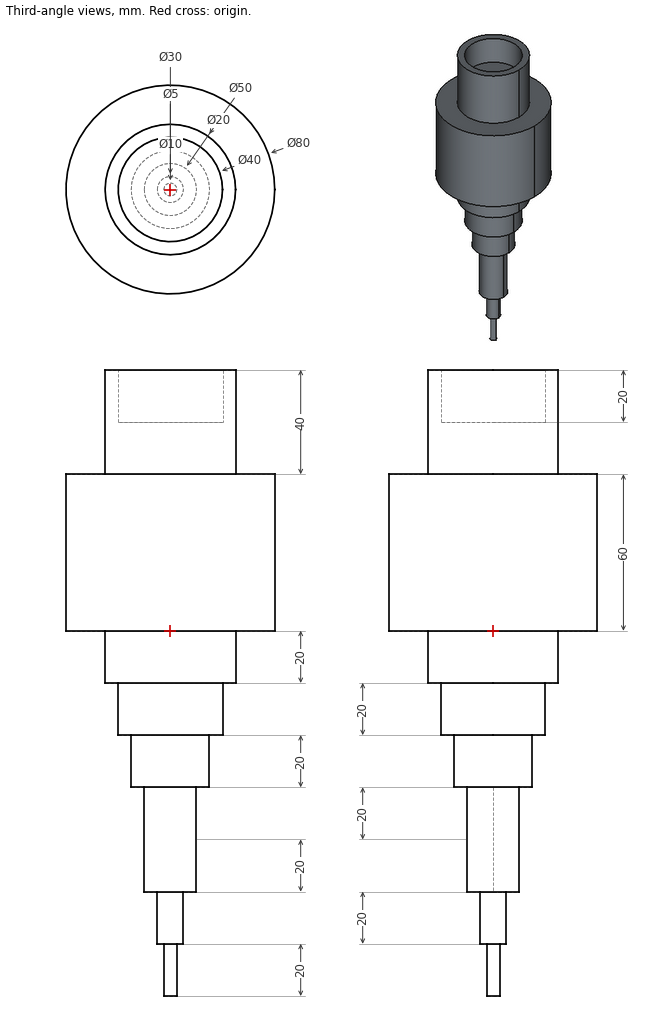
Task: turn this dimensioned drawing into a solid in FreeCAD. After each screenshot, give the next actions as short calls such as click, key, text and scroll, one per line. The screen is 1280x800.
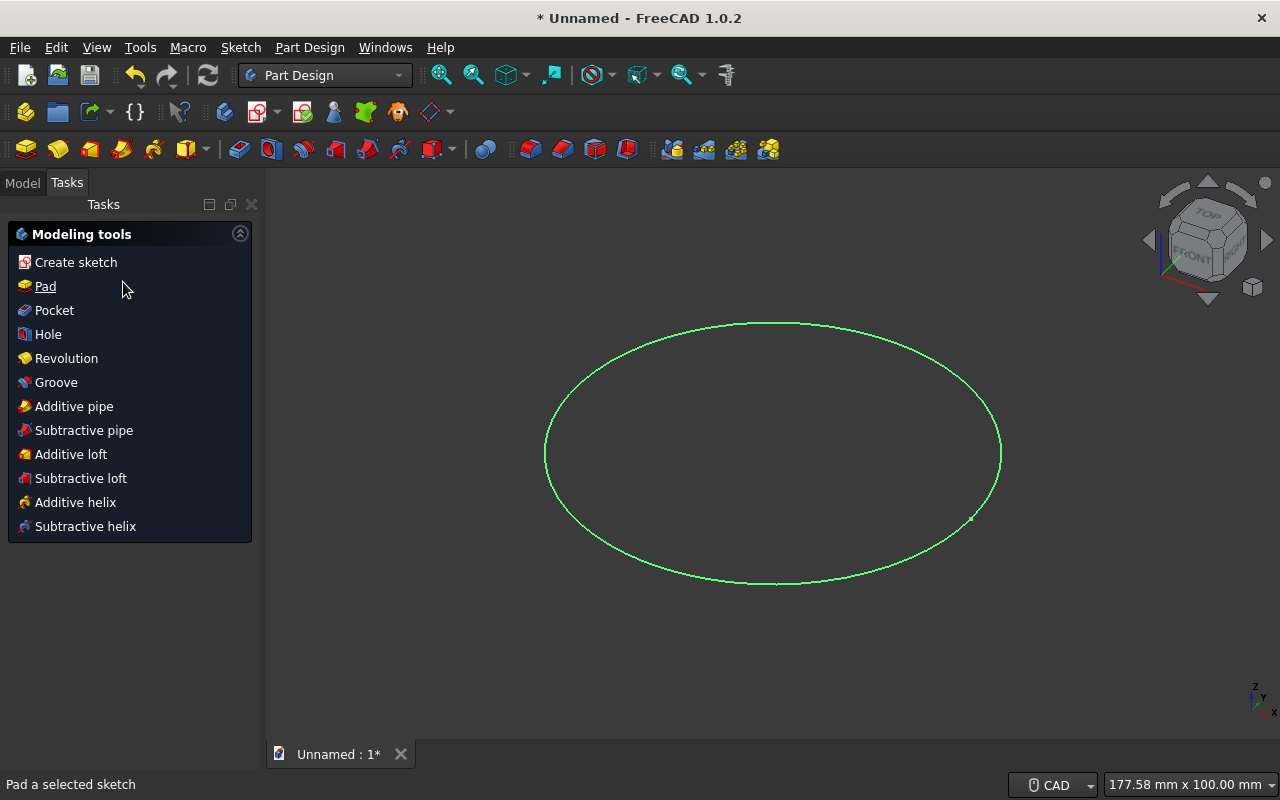
click(26, 150)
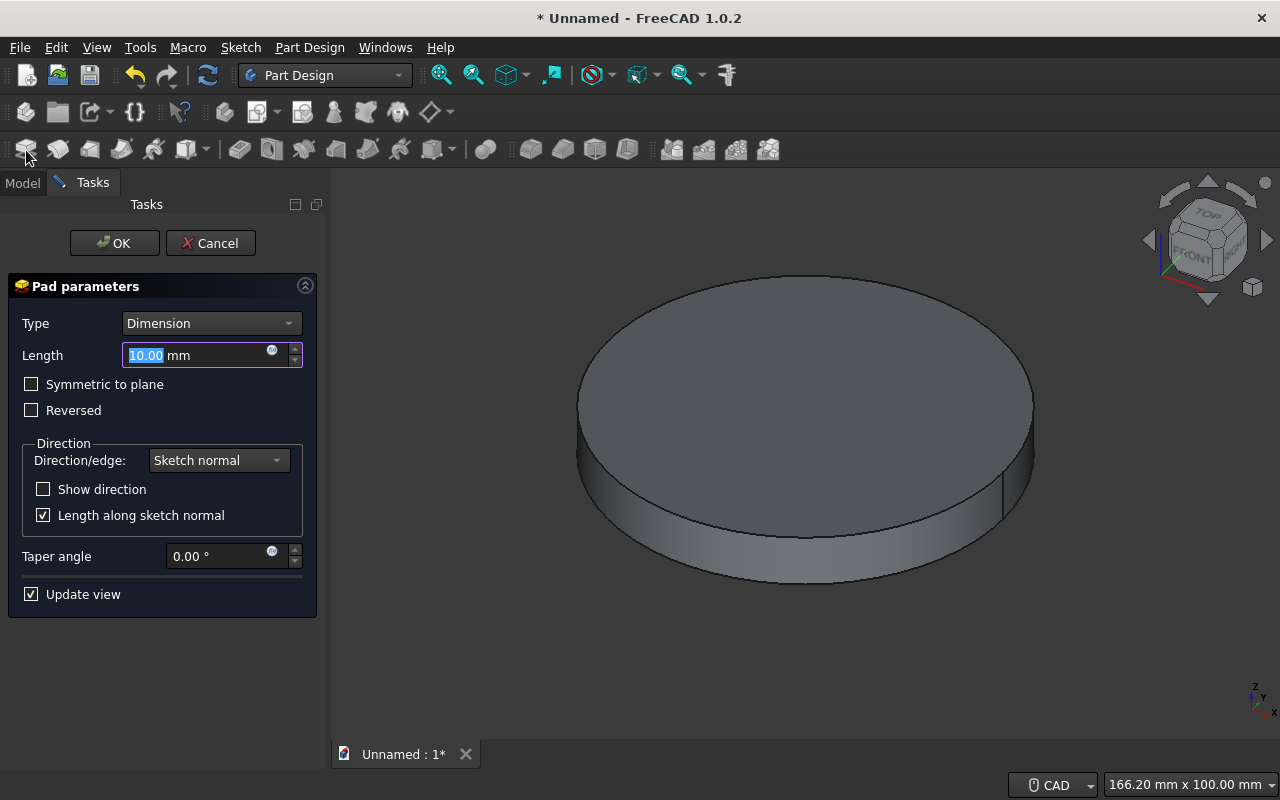
text(60)
key(Tab)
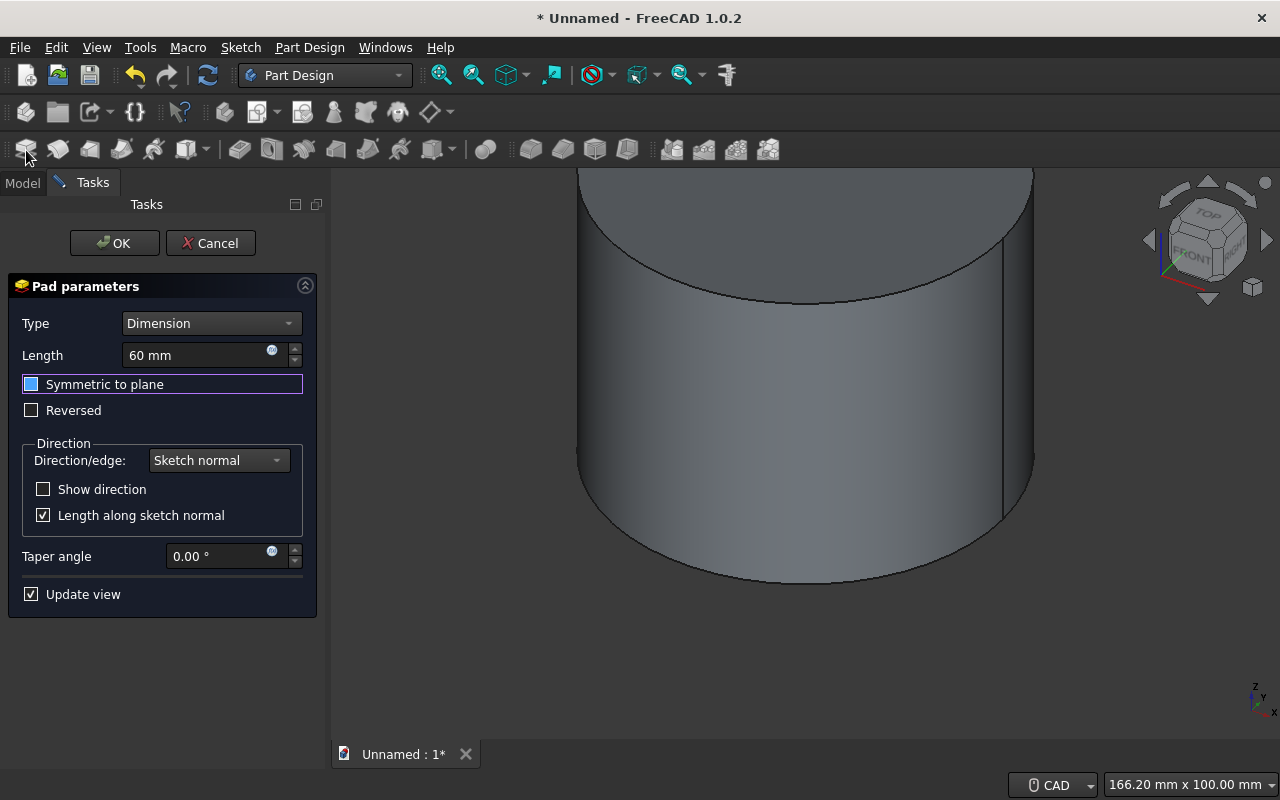
click(115, 243)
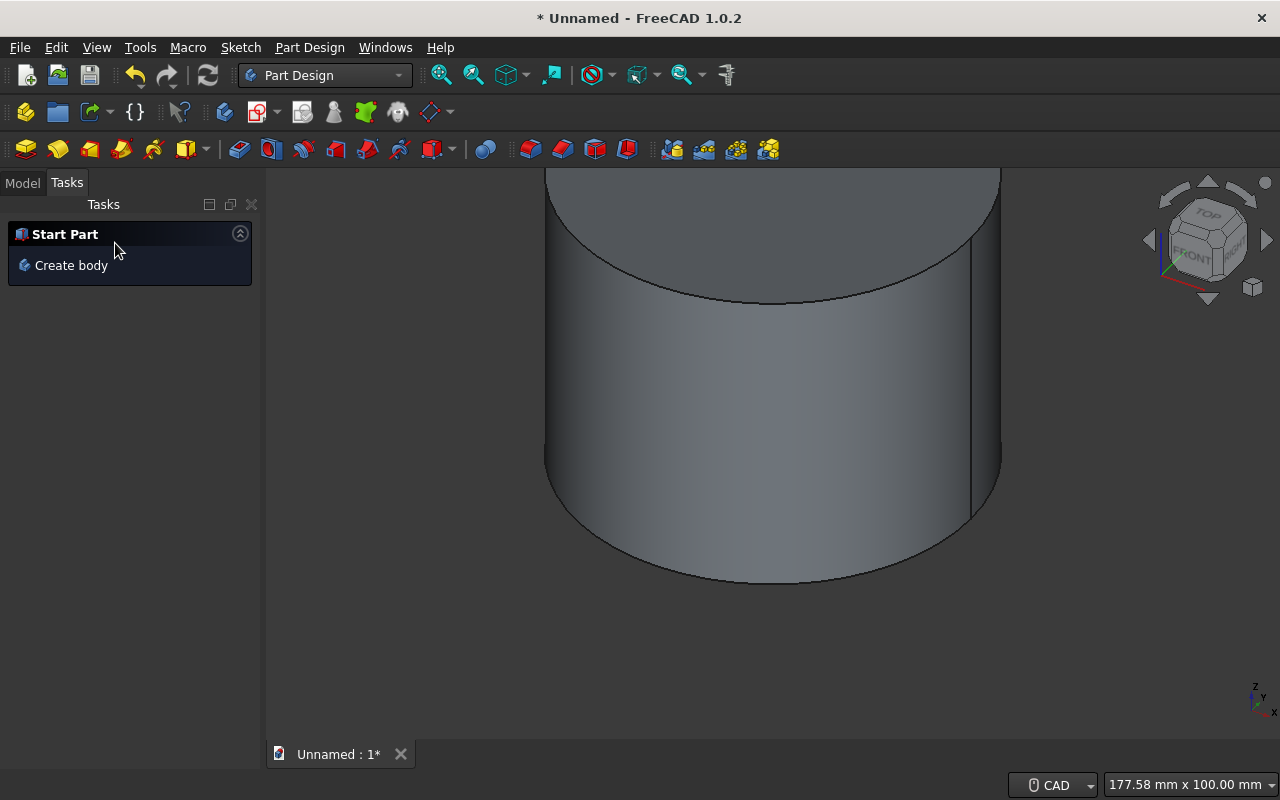
click(442, 76)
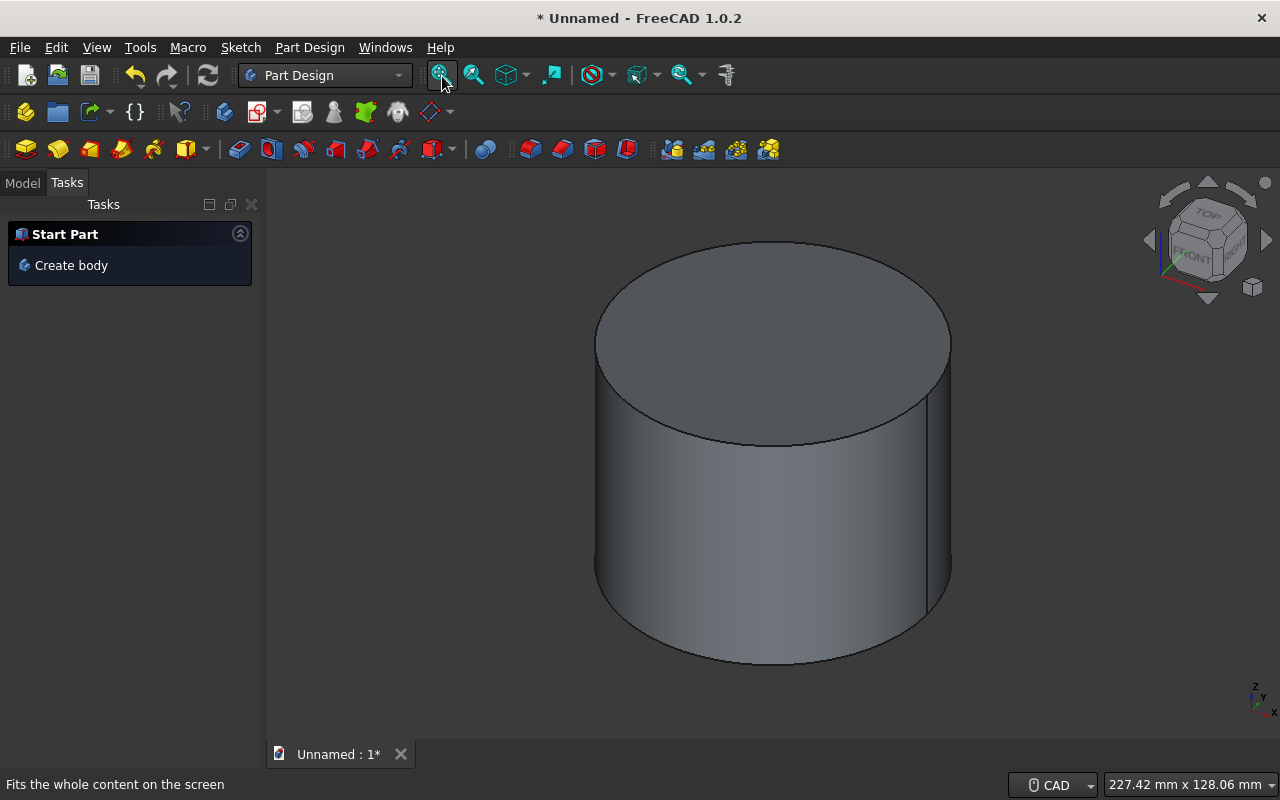
click(773, 343)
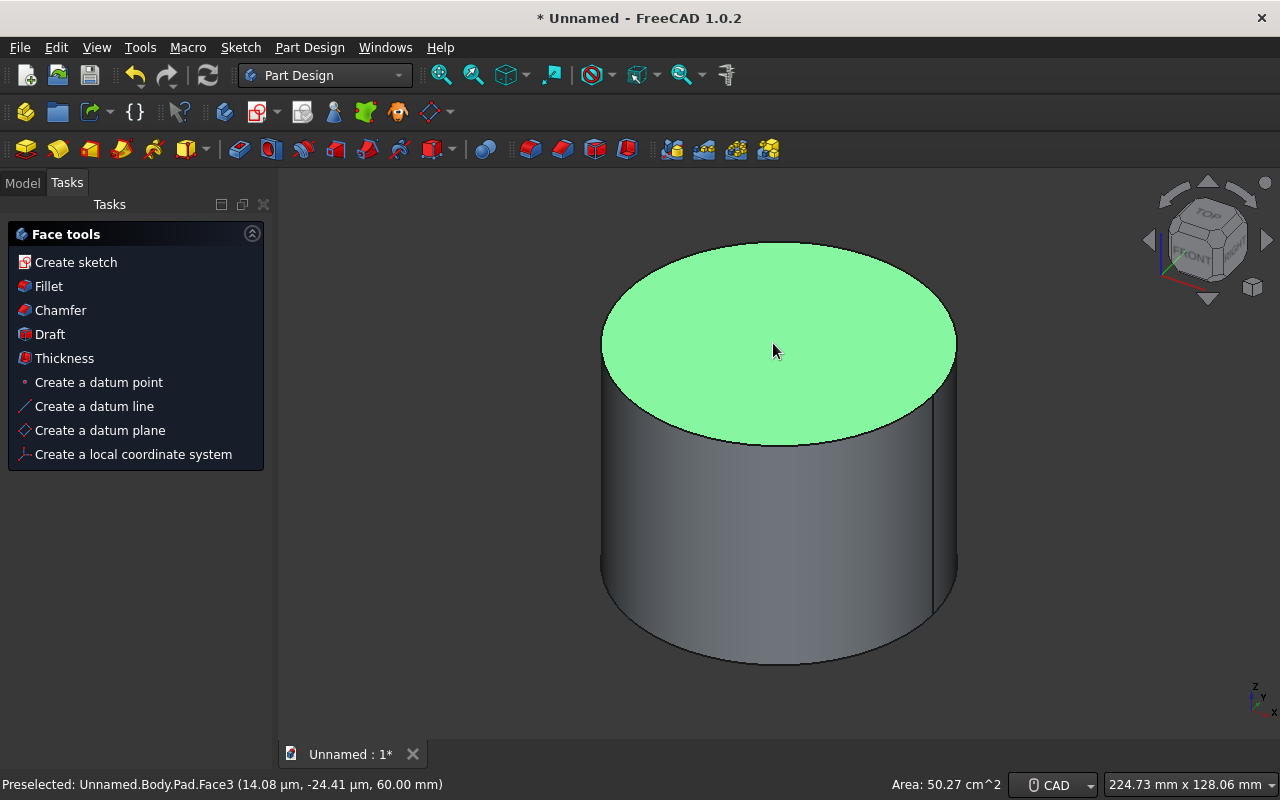
click(258, 112)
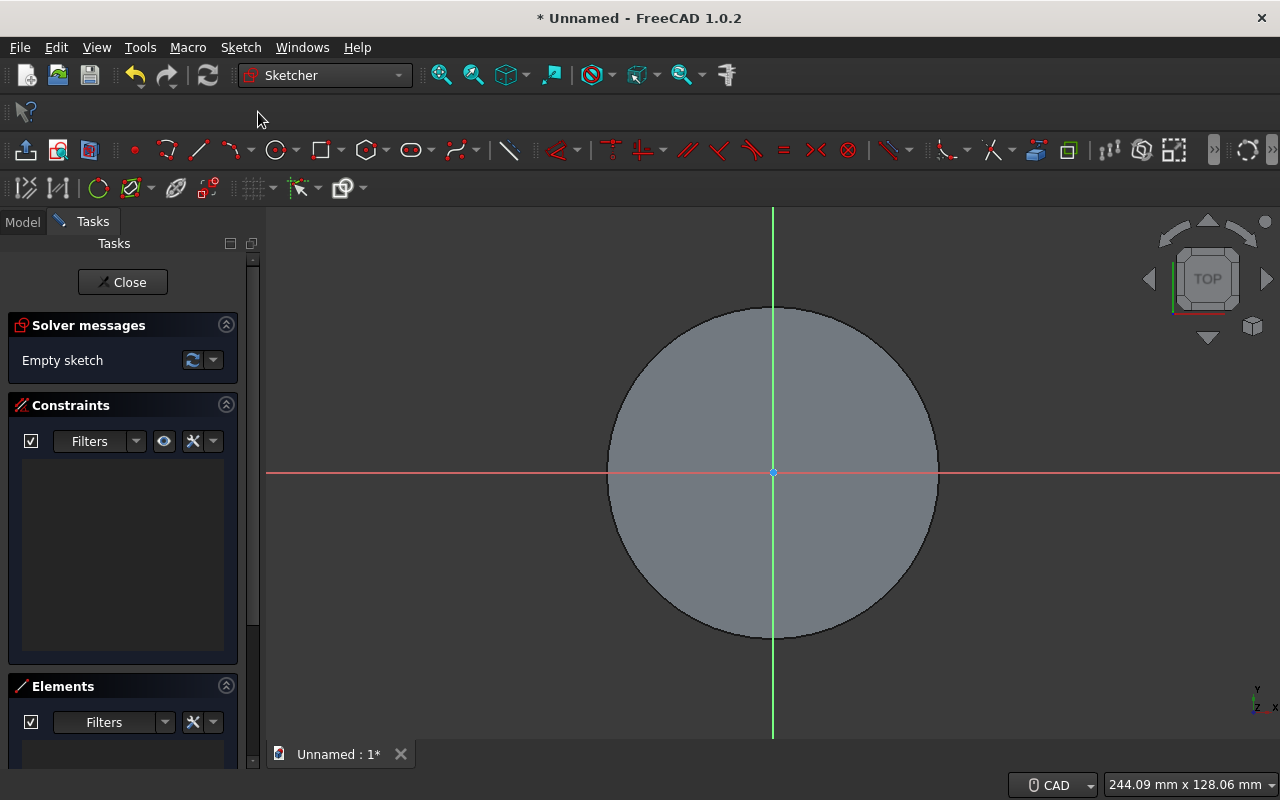
scroll(912, 473, up, 2)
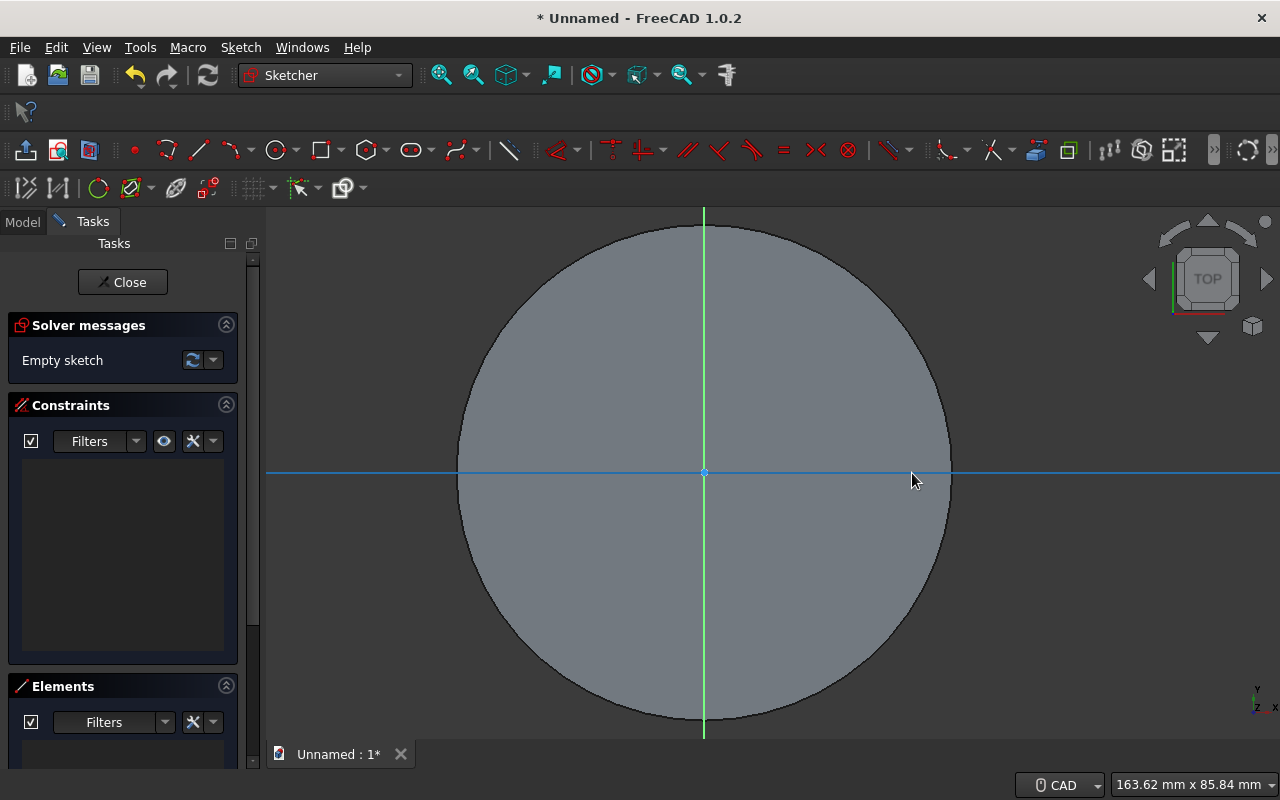
click(276, 150)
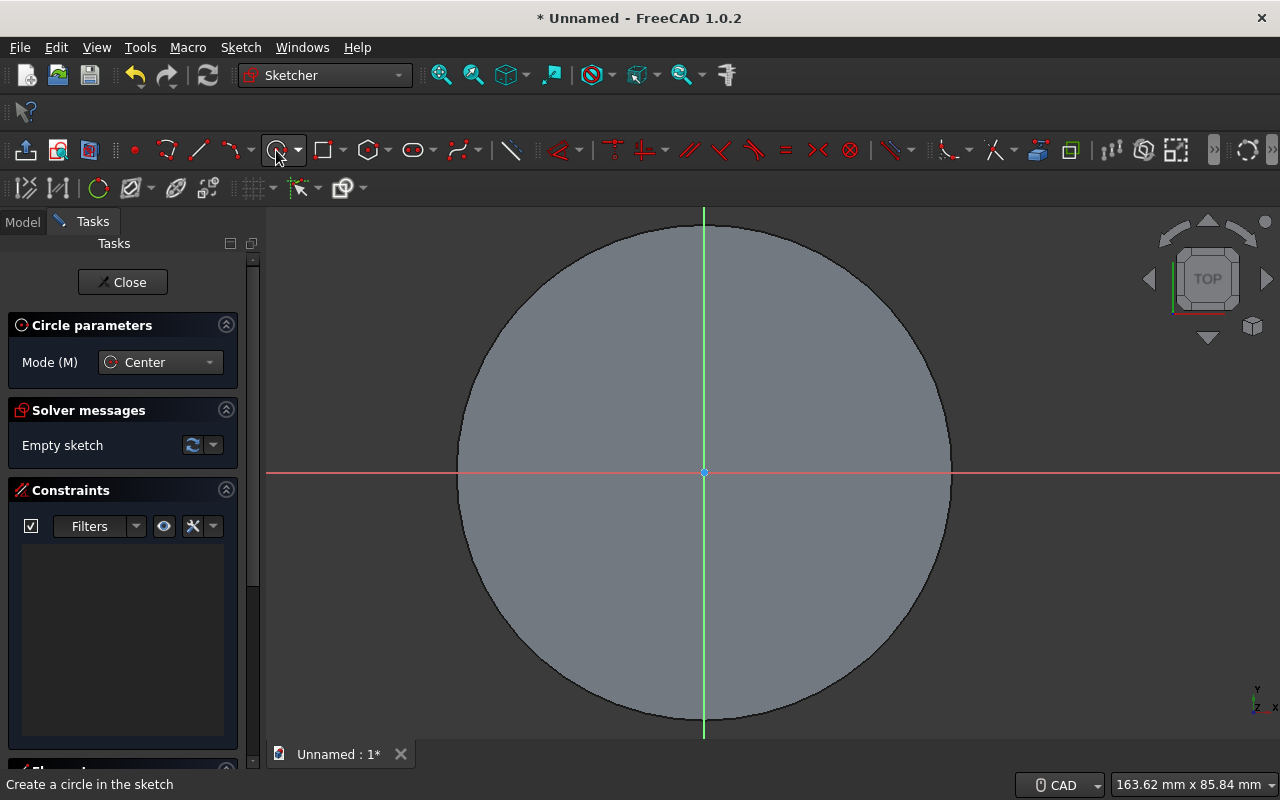
click(704, 473)
click(814, 363)
key(Escape)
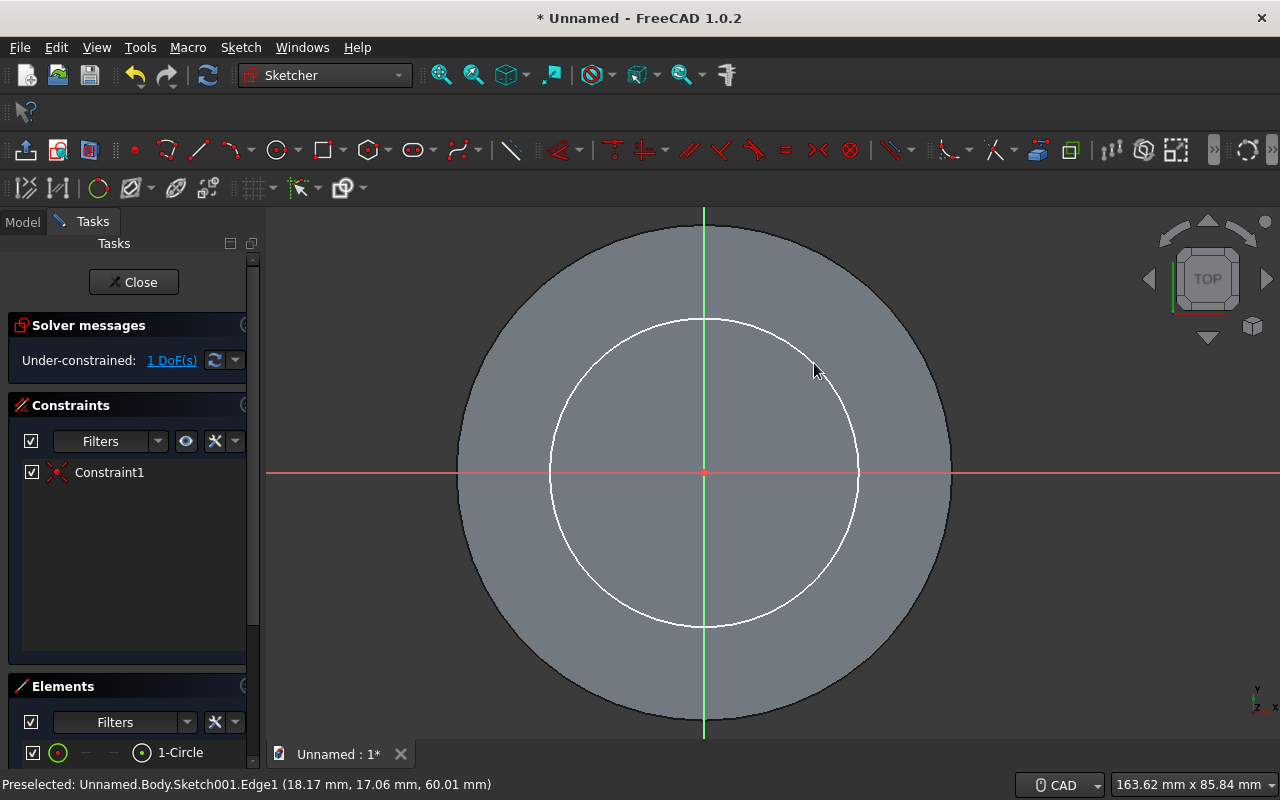
click(558, 150)